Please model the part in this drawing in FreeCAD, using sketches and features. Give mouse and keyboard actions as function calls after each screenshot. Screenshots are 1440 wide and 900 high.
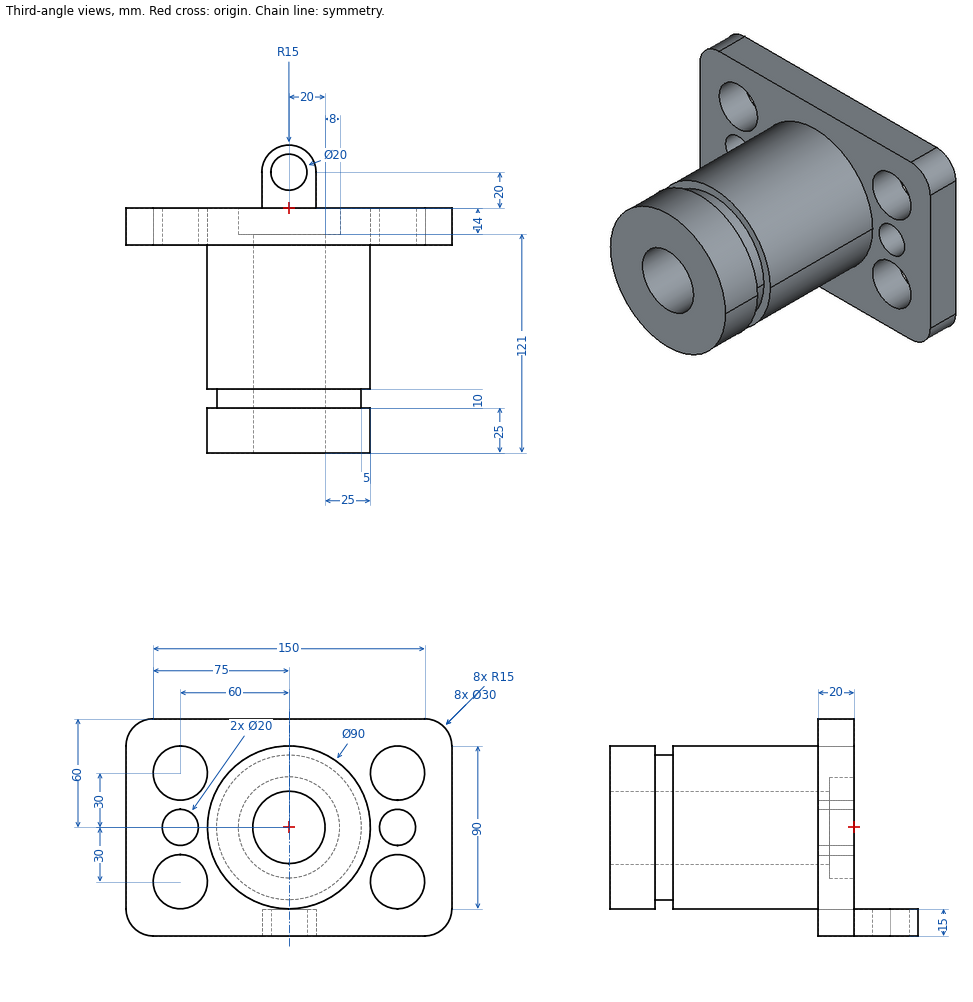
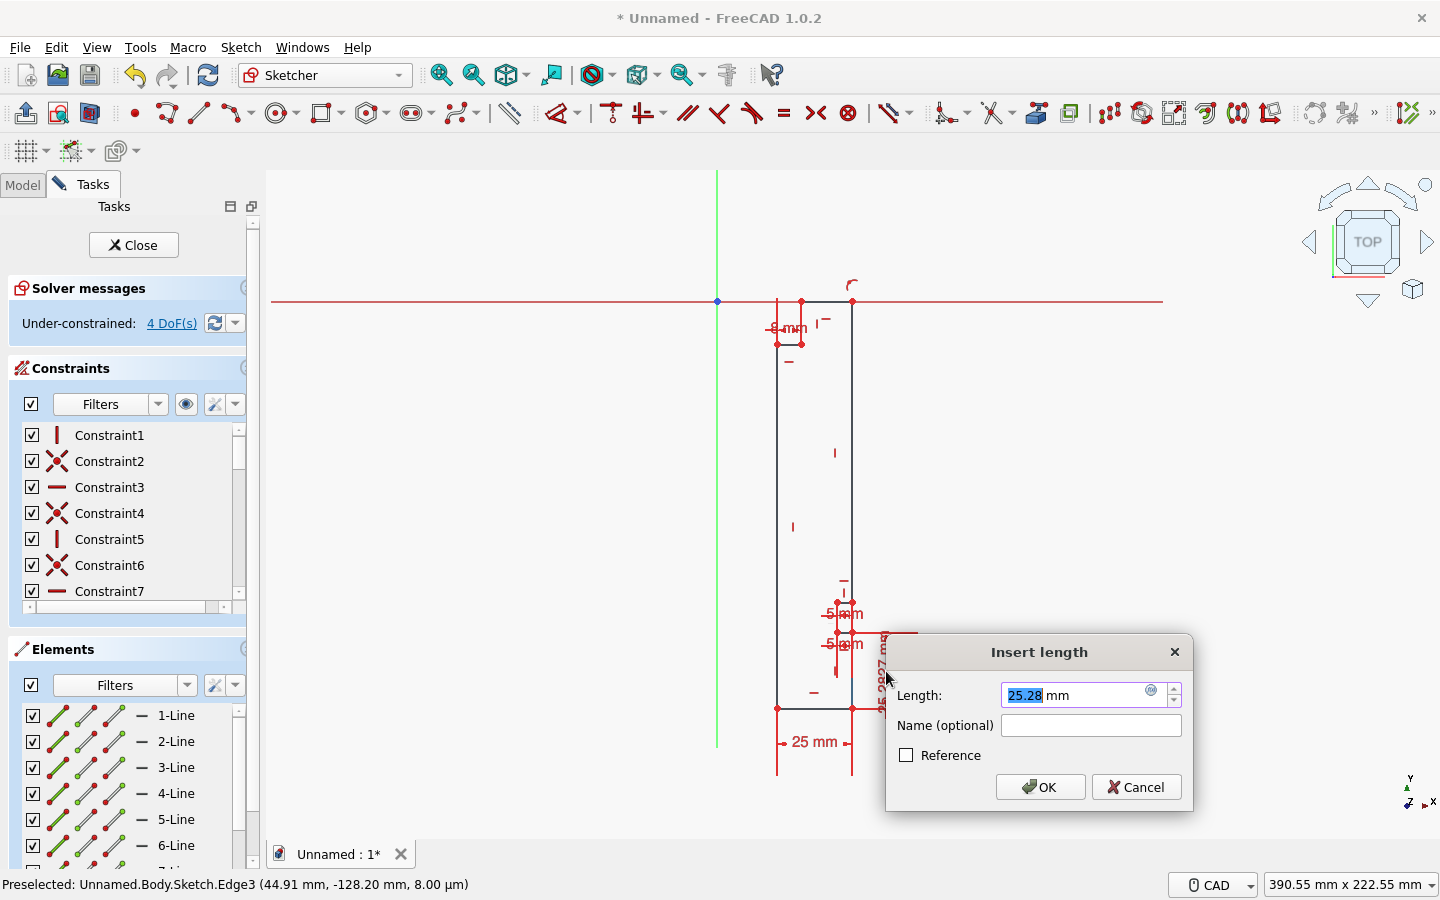
text(25)
key(Return)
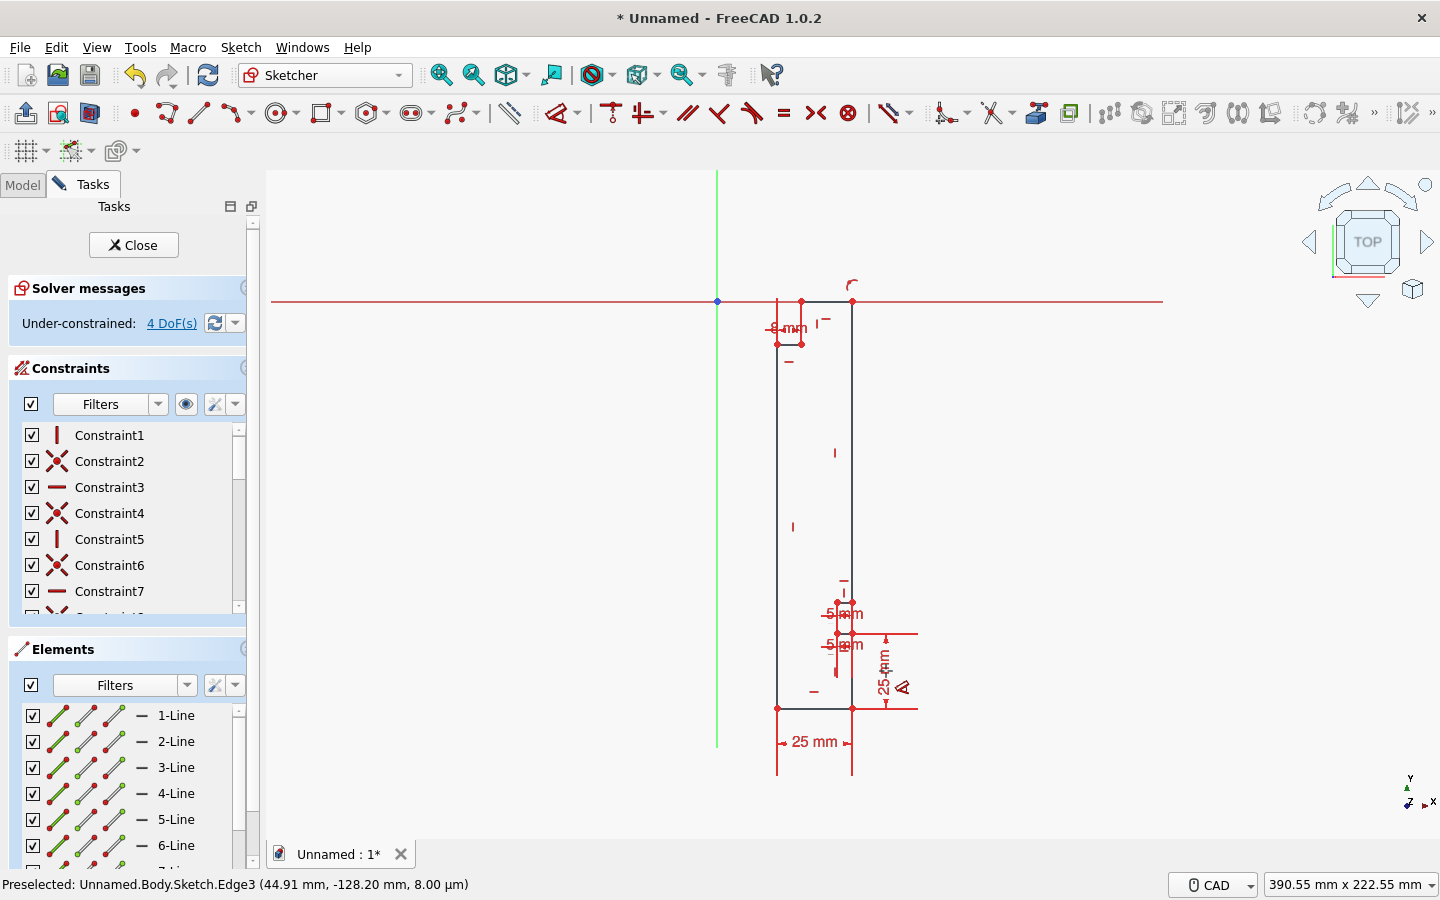
scroll(837, 624, up, 3)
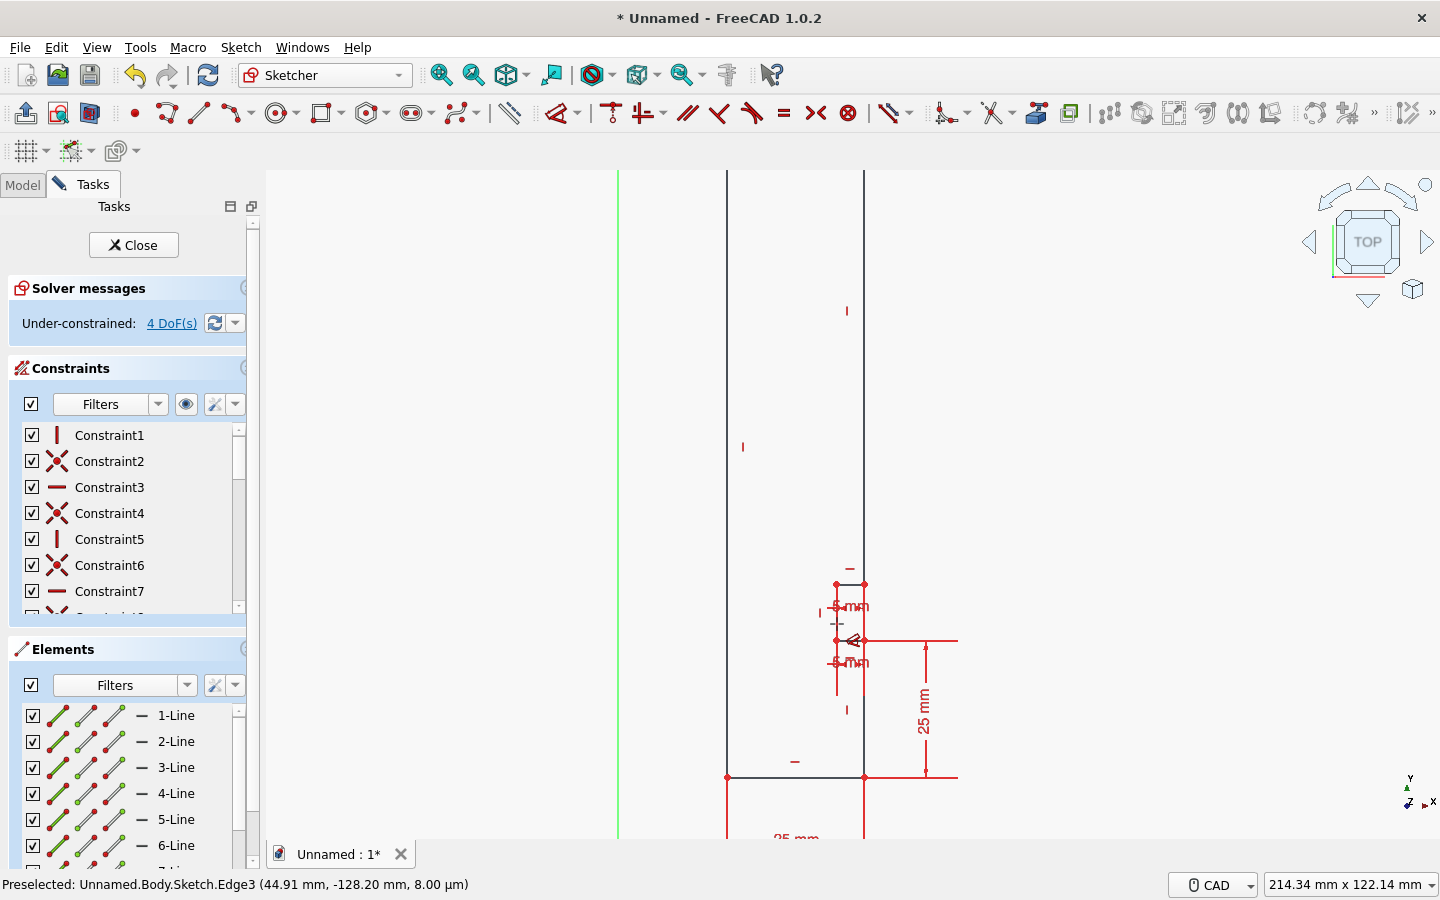
click(837, 624)
click(803, 632)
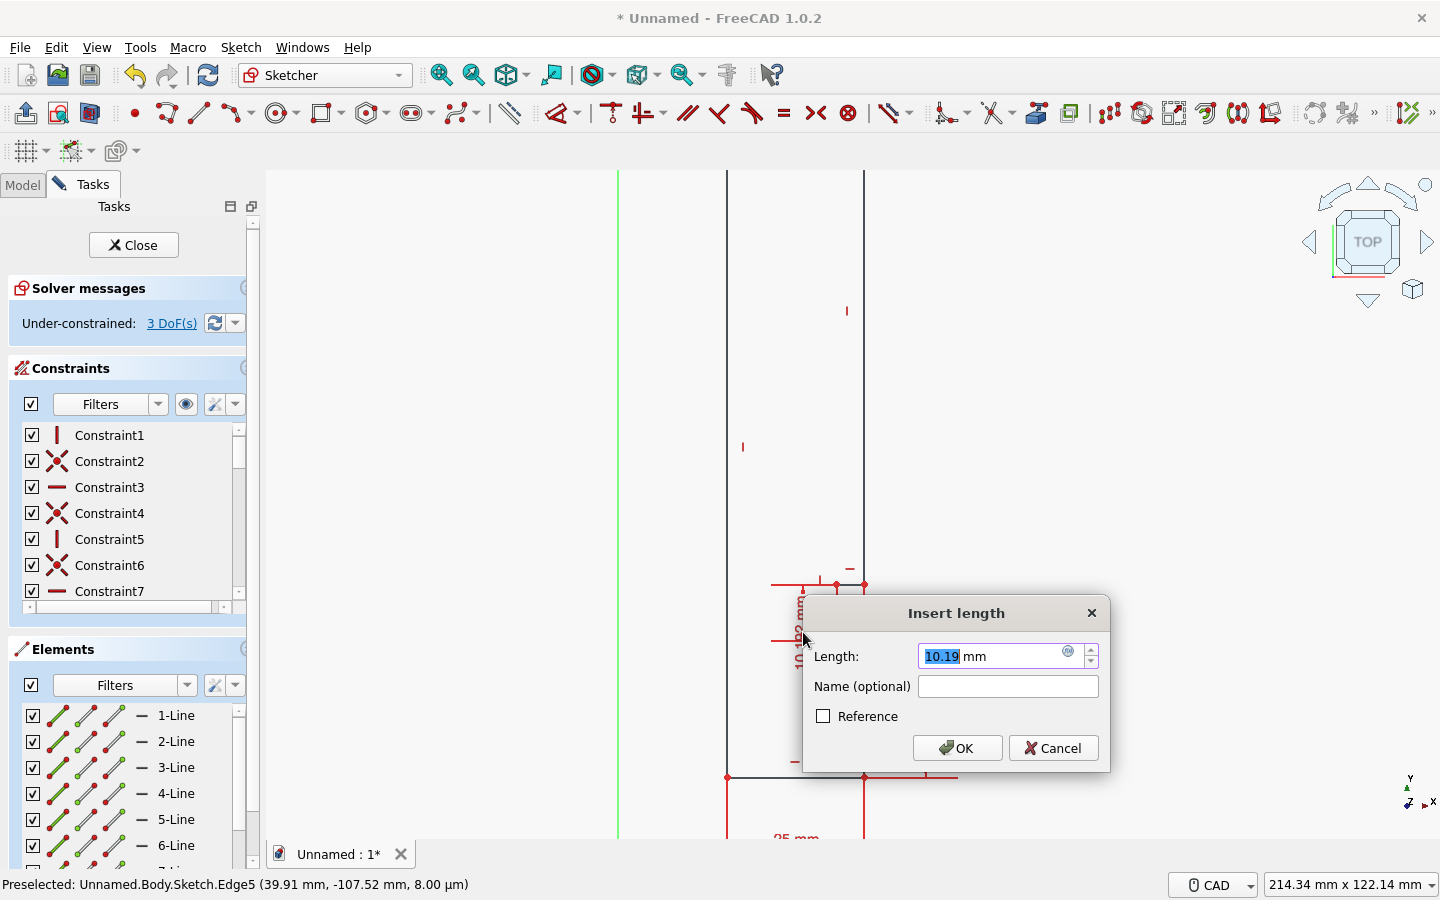
text(10)
key(Return)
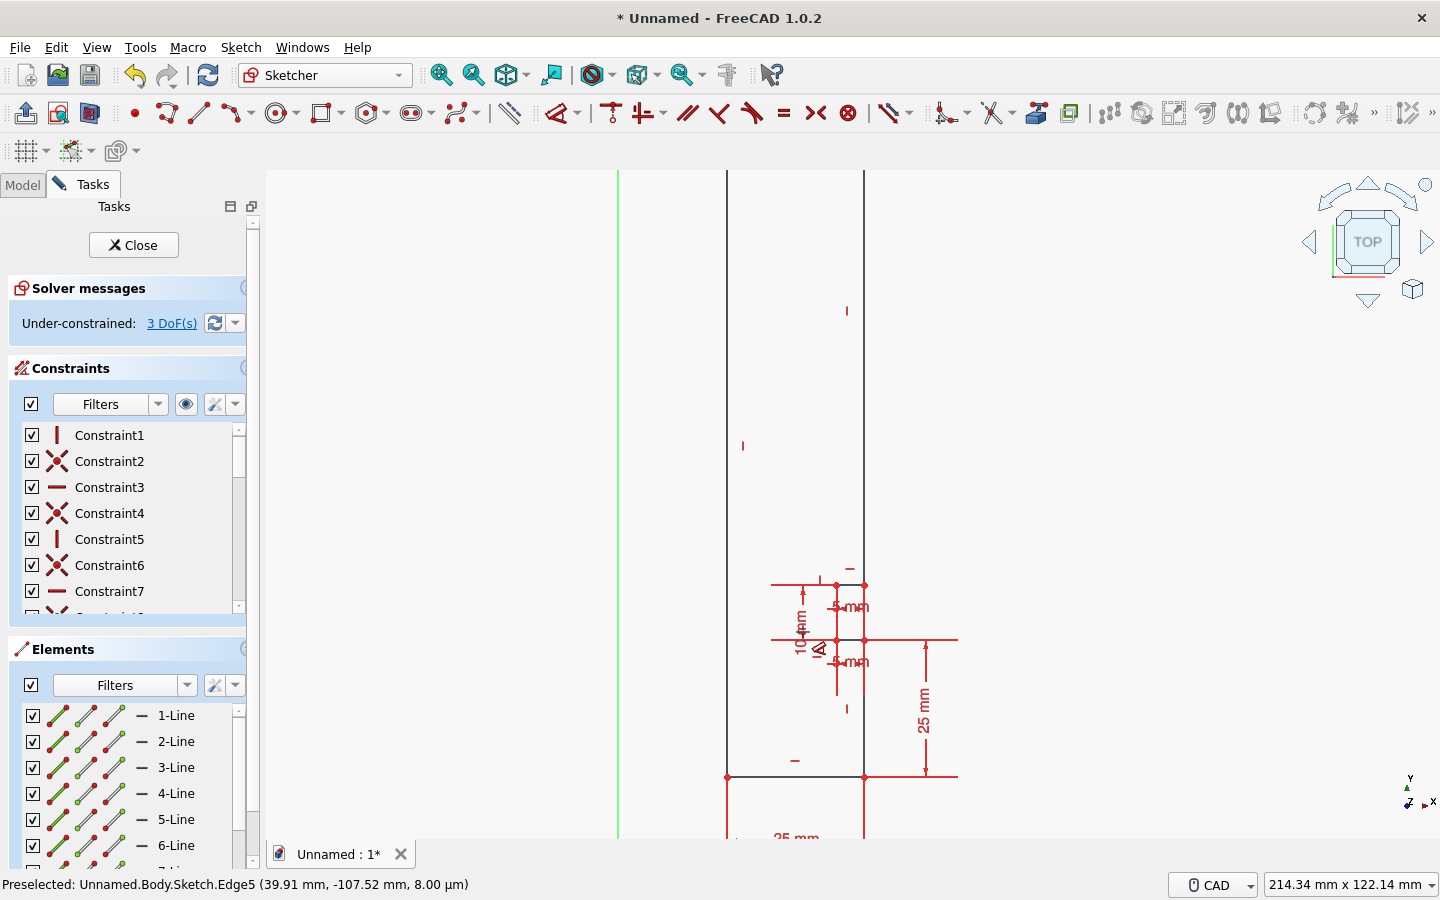
scroll(837, 625, down, 3)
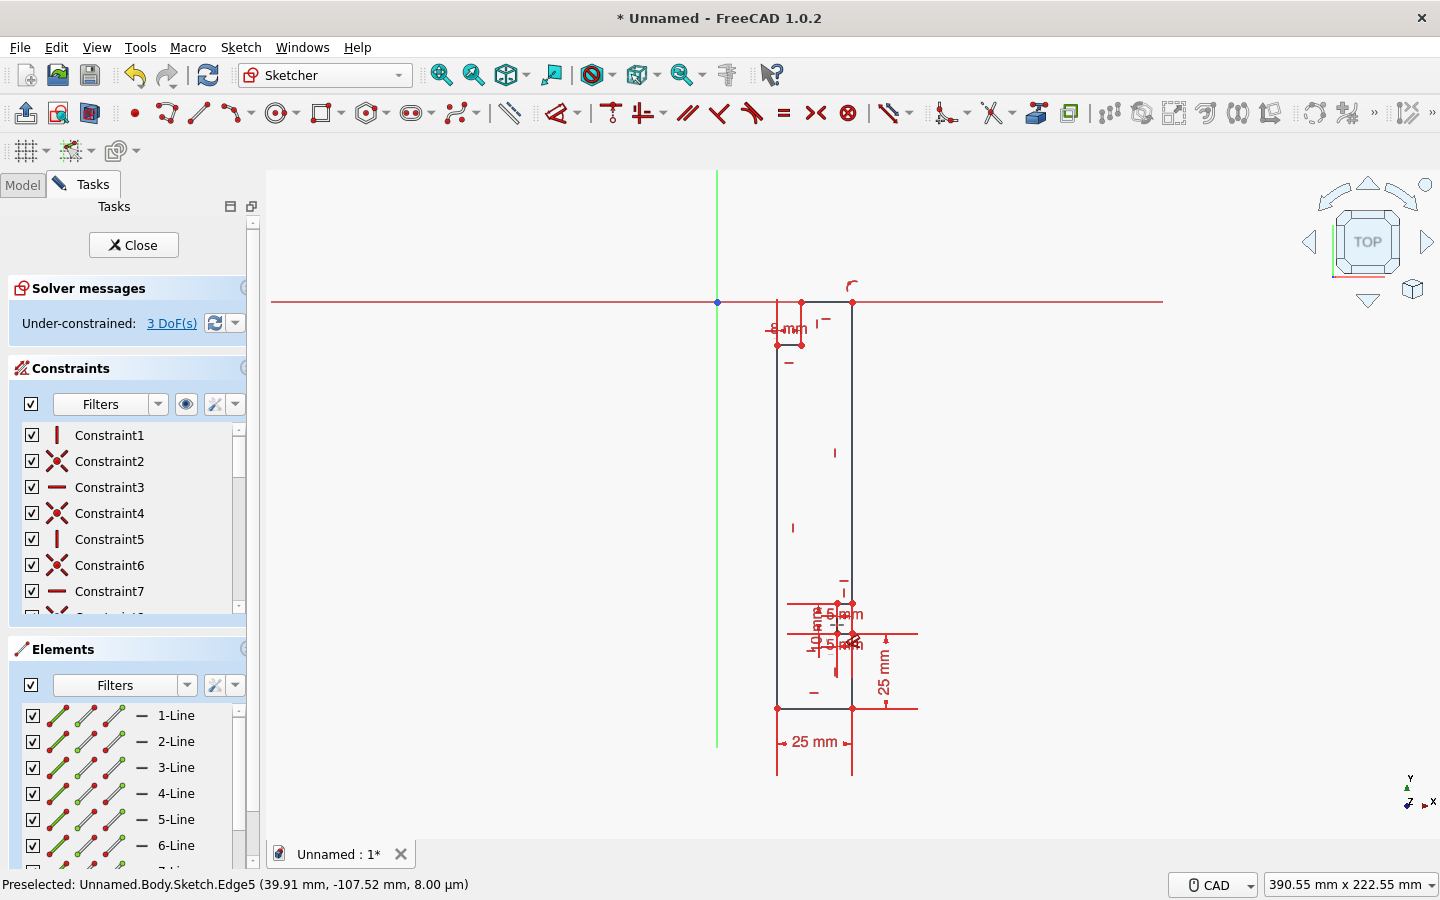
click(801, 315)
click(883, 324)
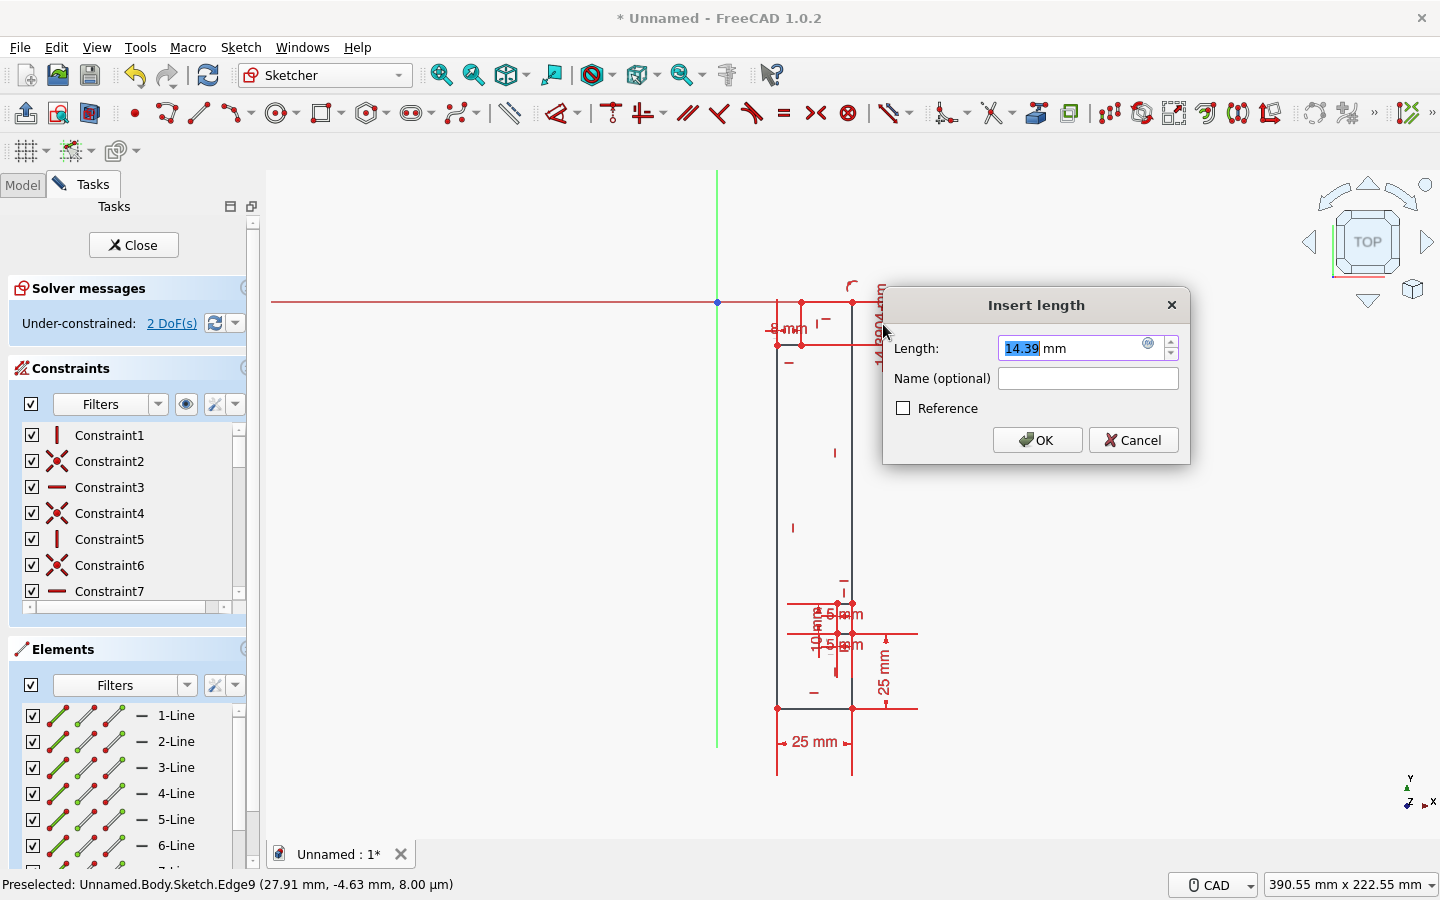
text(14)
key(Return)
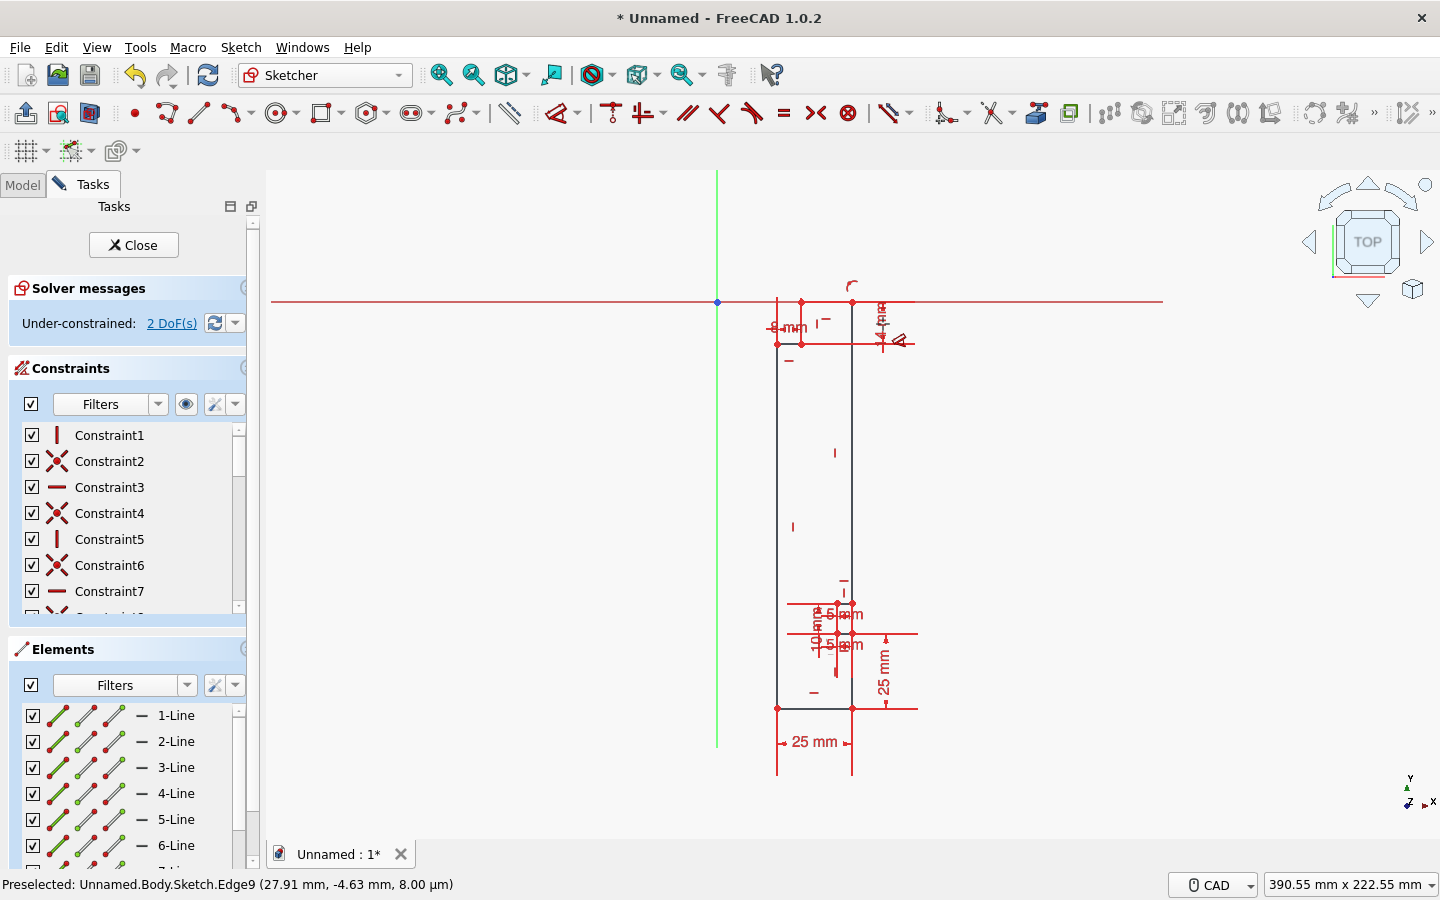
click(777, 454)
click(743, 526)